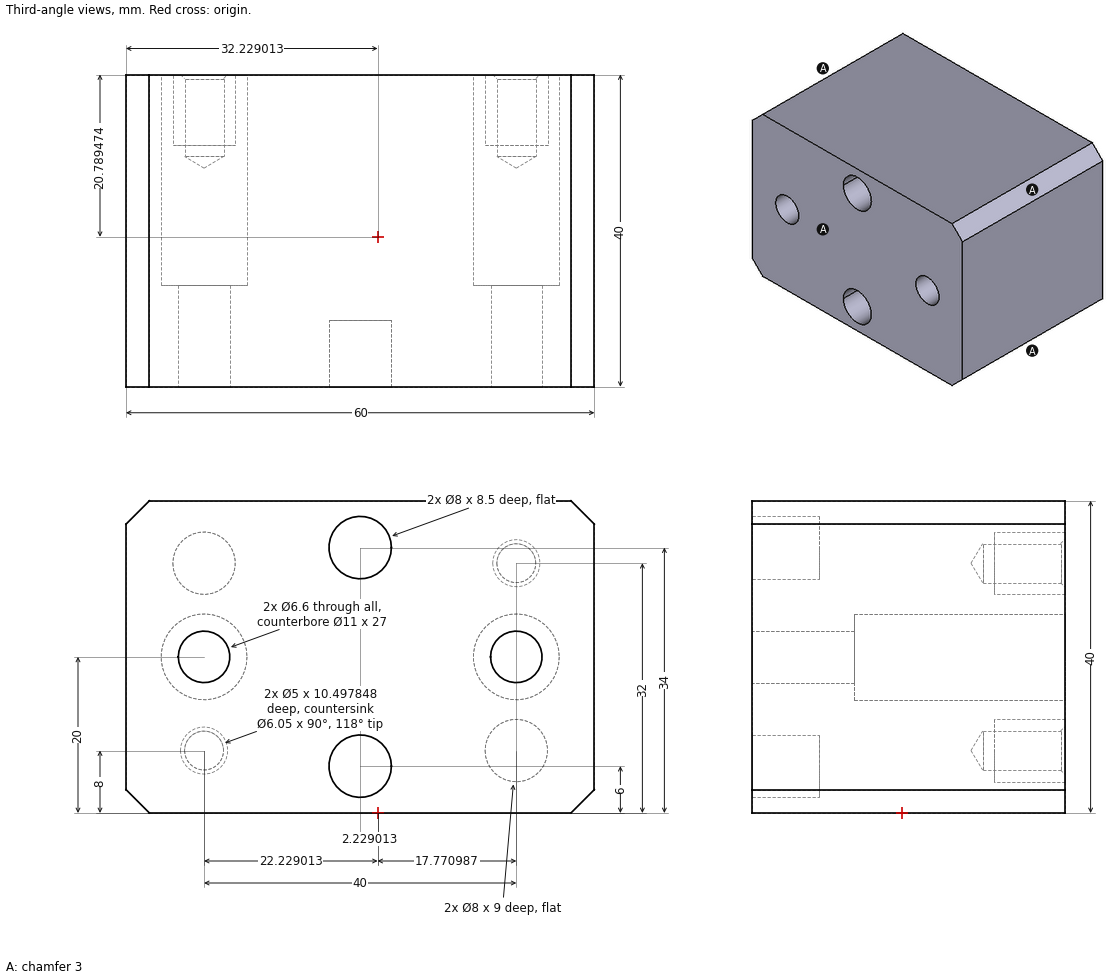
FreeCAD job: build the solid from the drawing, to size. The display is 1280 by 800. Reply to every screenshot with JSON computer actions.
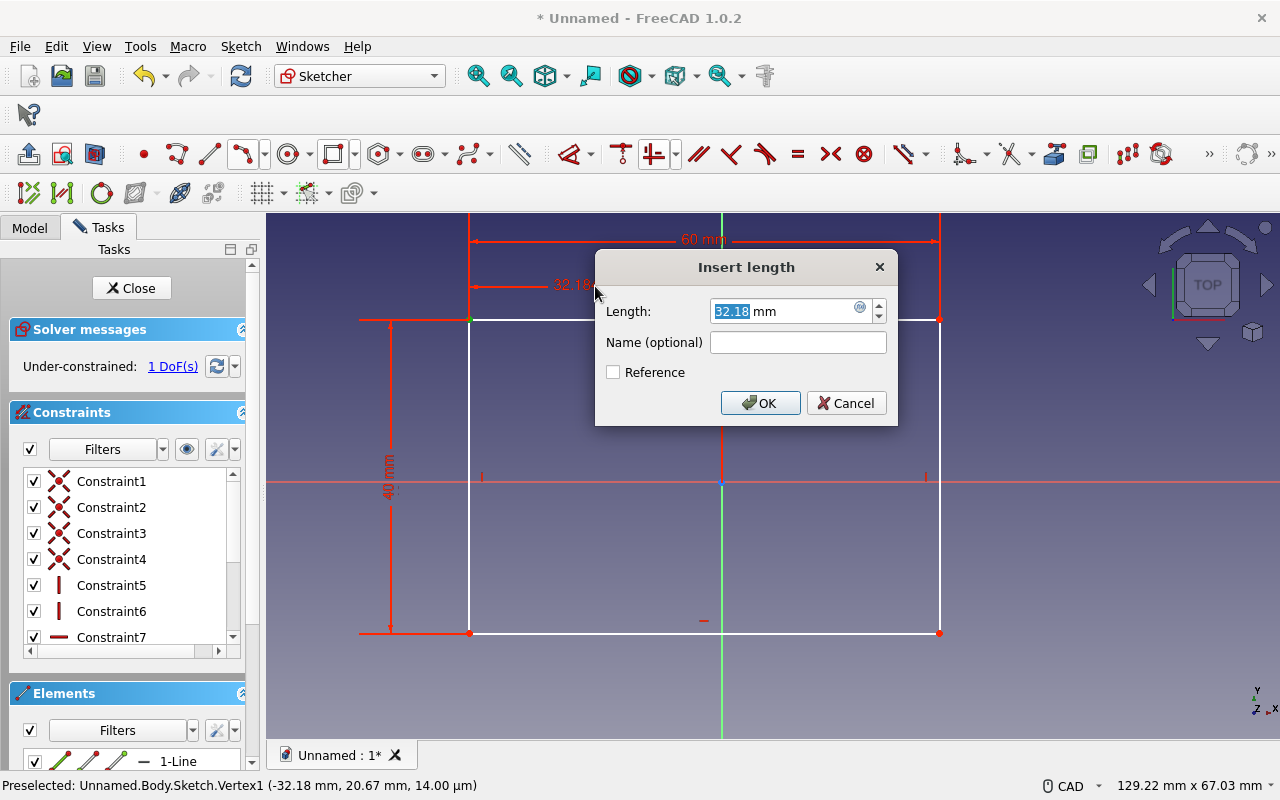
{"action": "type", "text": "32.229013"}
{"action": "key", "text": "Return"}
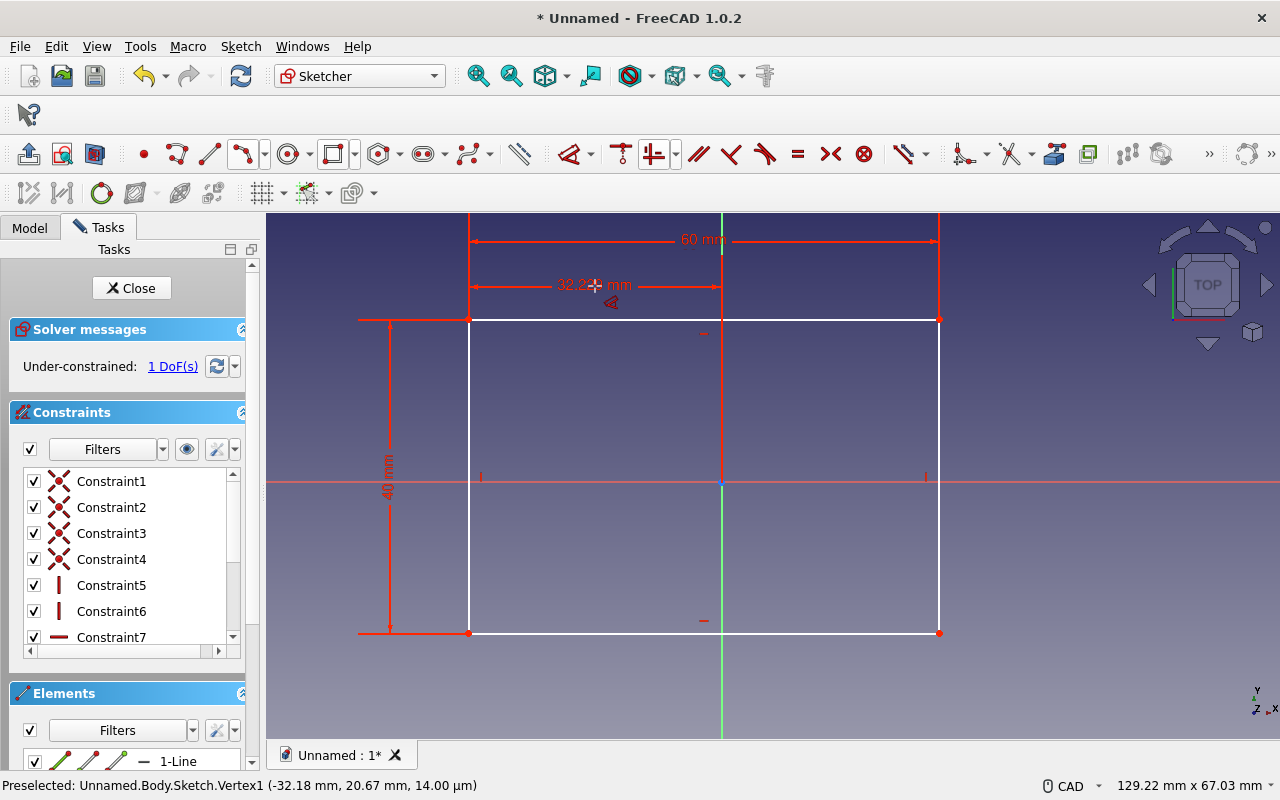
{"action": "left_click", "coordinate": [469, 320]}
{"action": "left_click", "coordinate": [435, 401]}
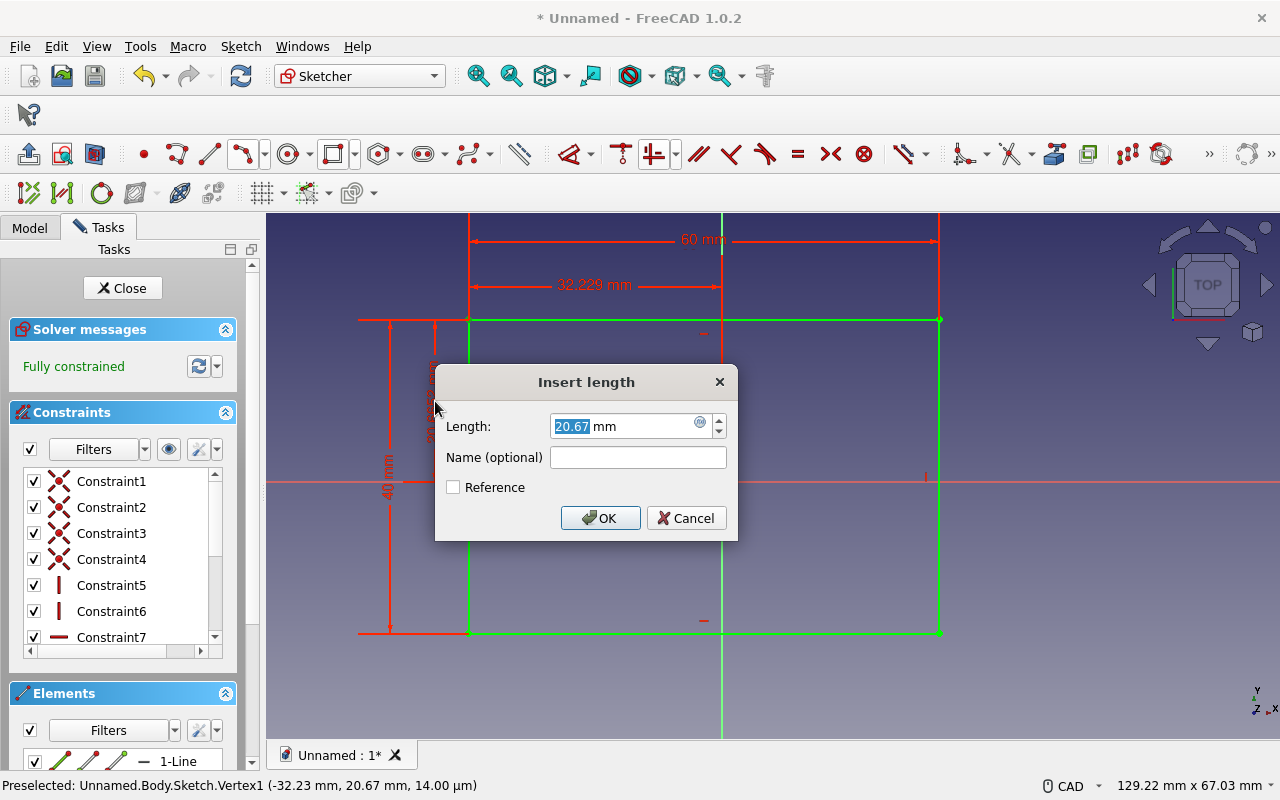
{"action": "type", "text": "20.789474"}
{"action": "key", "text": "Return"}
{"action": "key", "text": "Escape"}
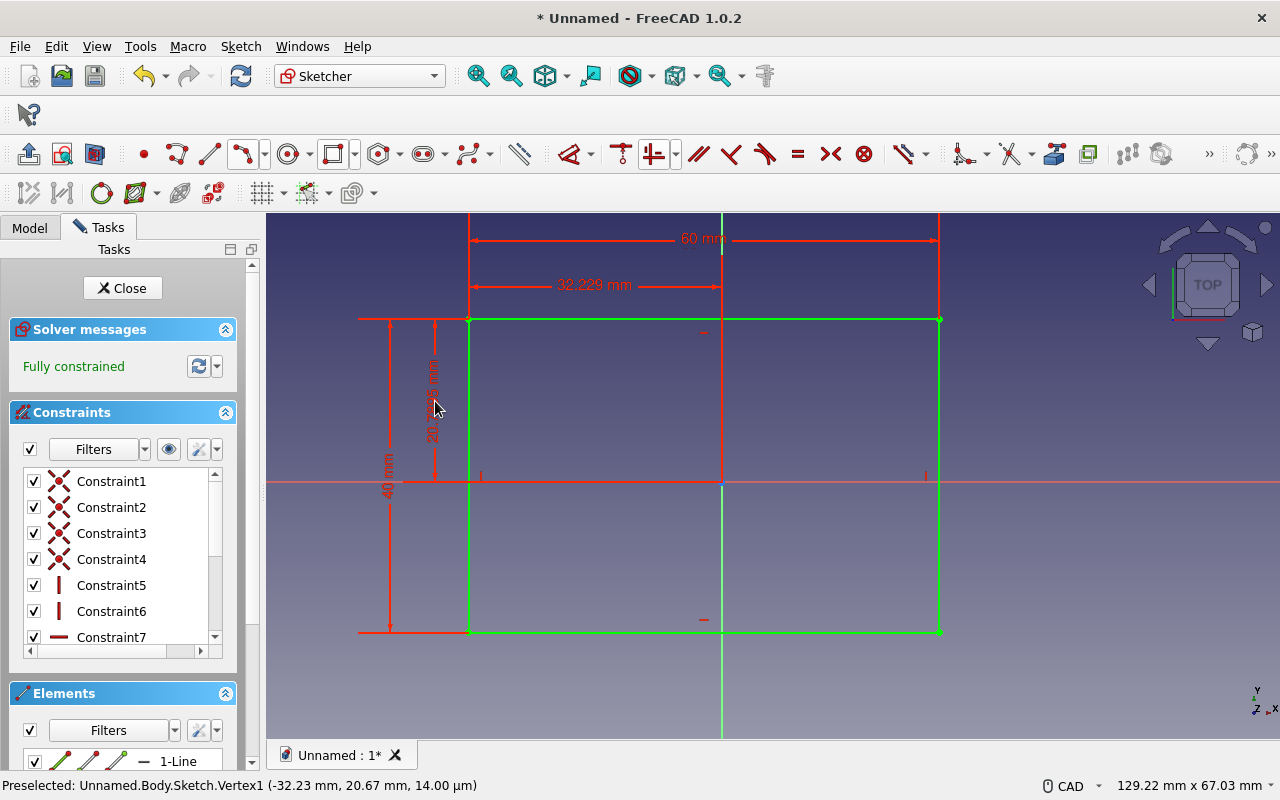
{"action": "left_click", "coordinate": [123, 288]}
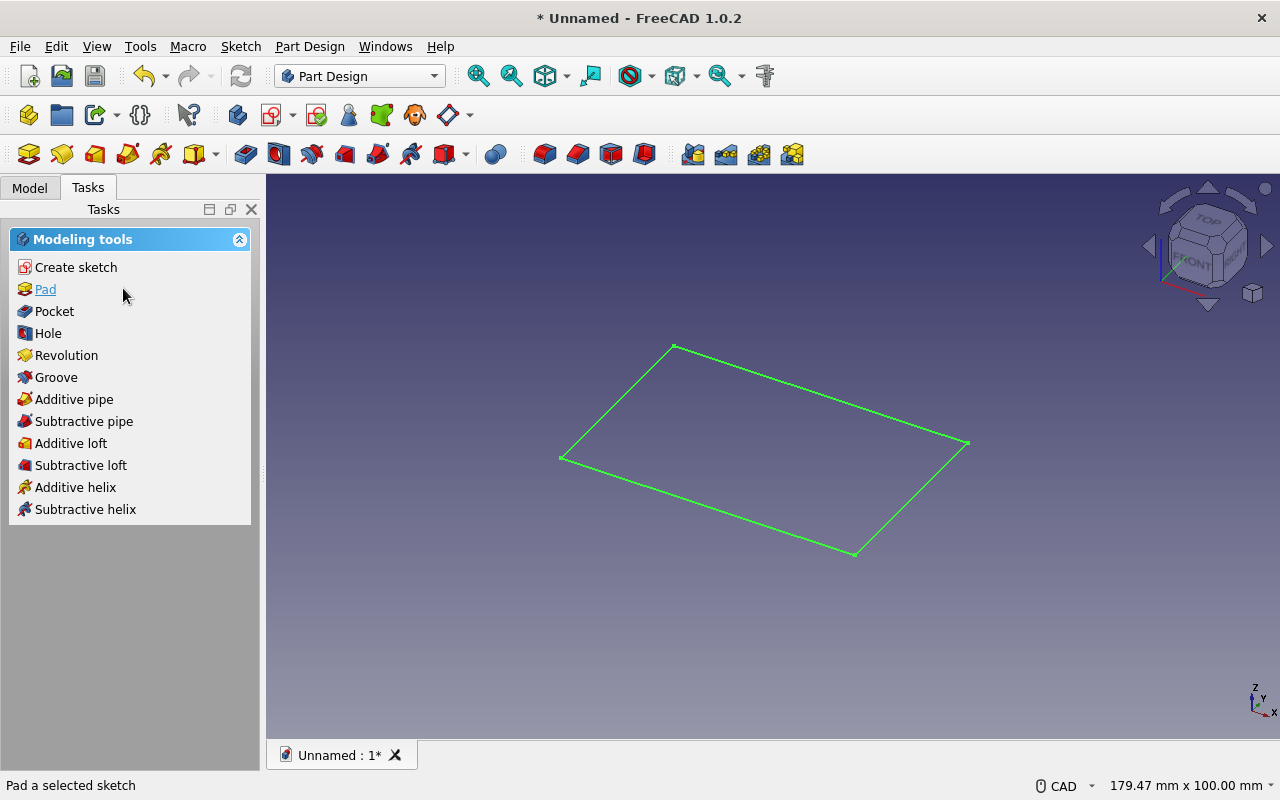
{"action": "left_click", "coordinate": [29, 154]}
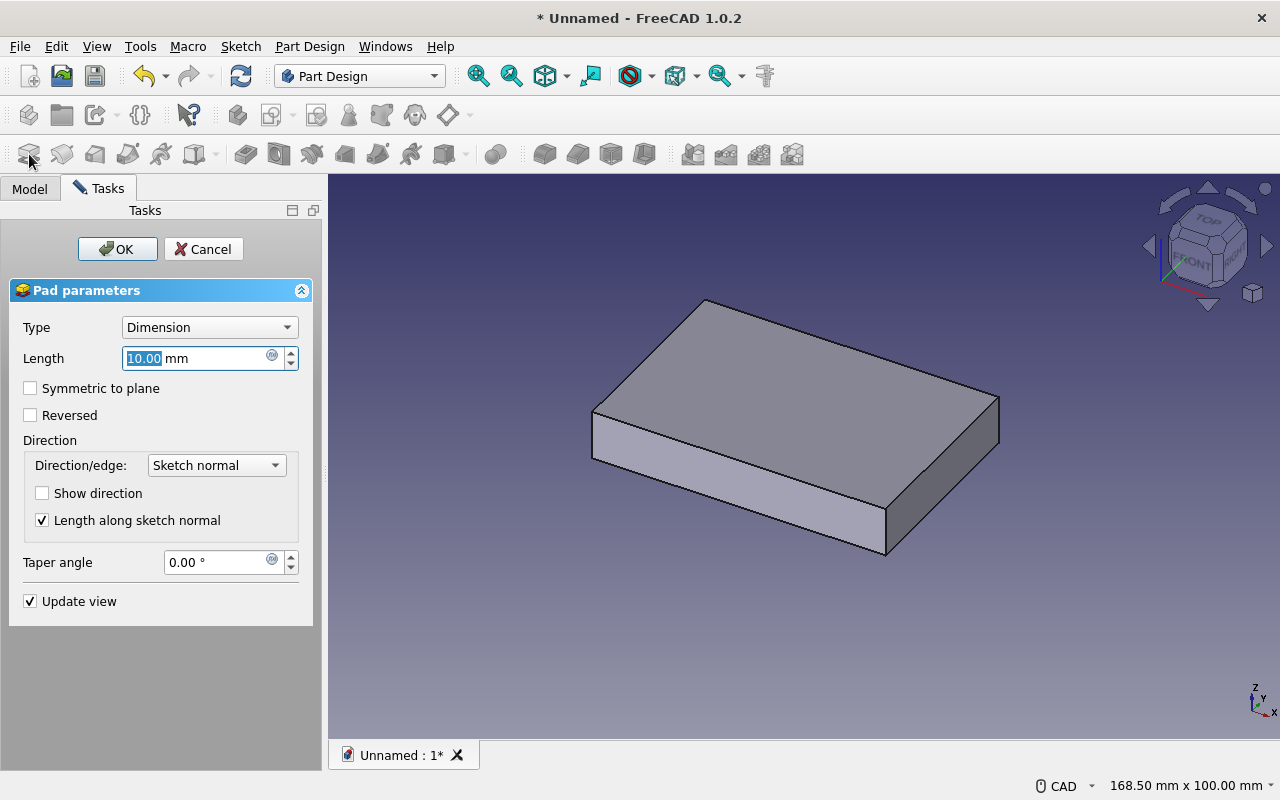
{"action": "type", "text": "40"}
{"action": "key", "text": "Tab"}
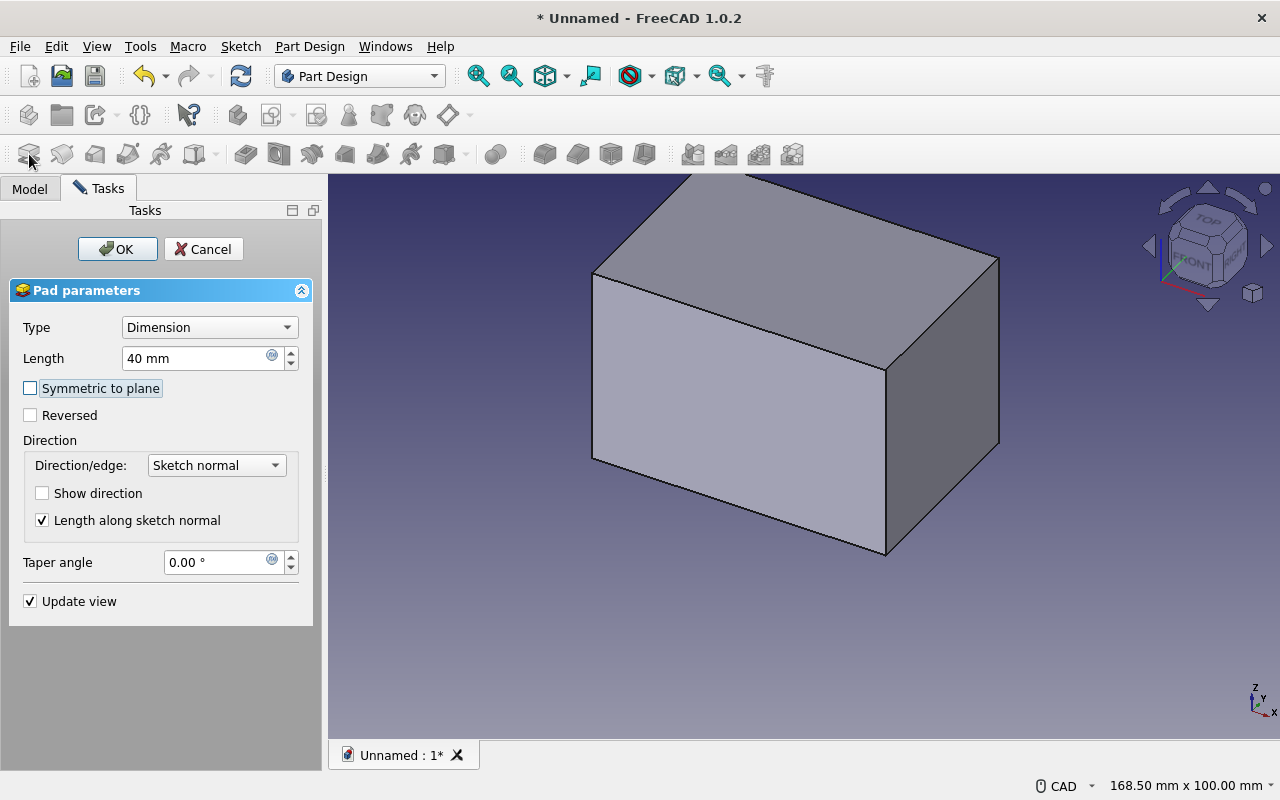
{"action": "left_click", "coordinate": [118, 249]}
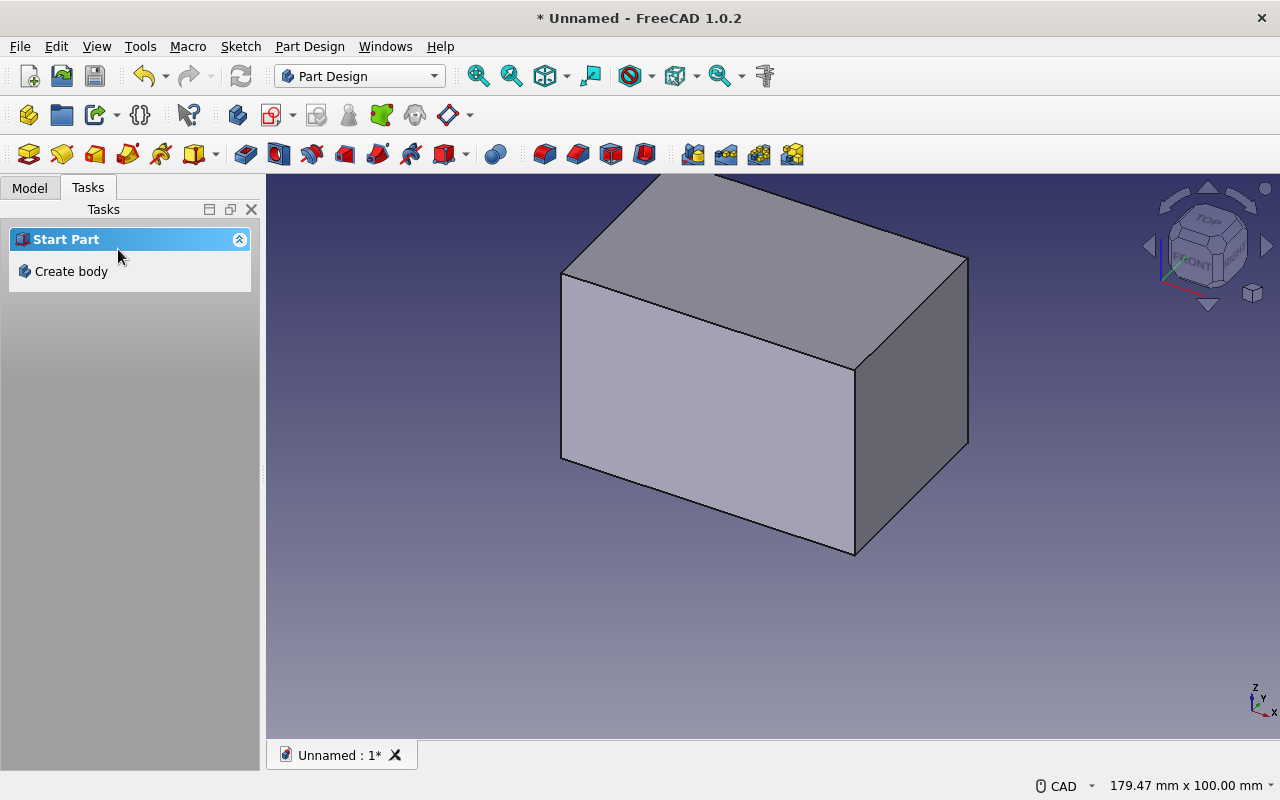
{"action": "key", "text": "v f"}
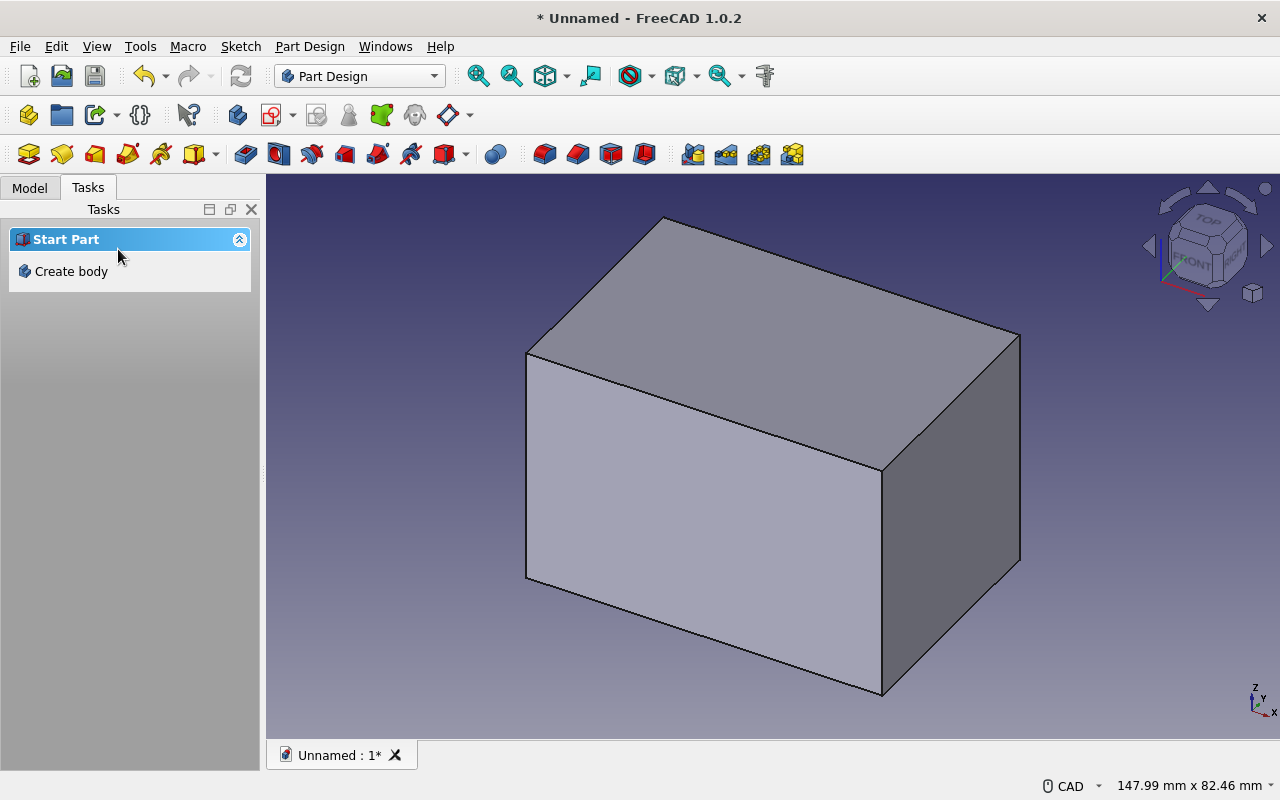
{"action": "left_click", "coordinate": [951, 402]}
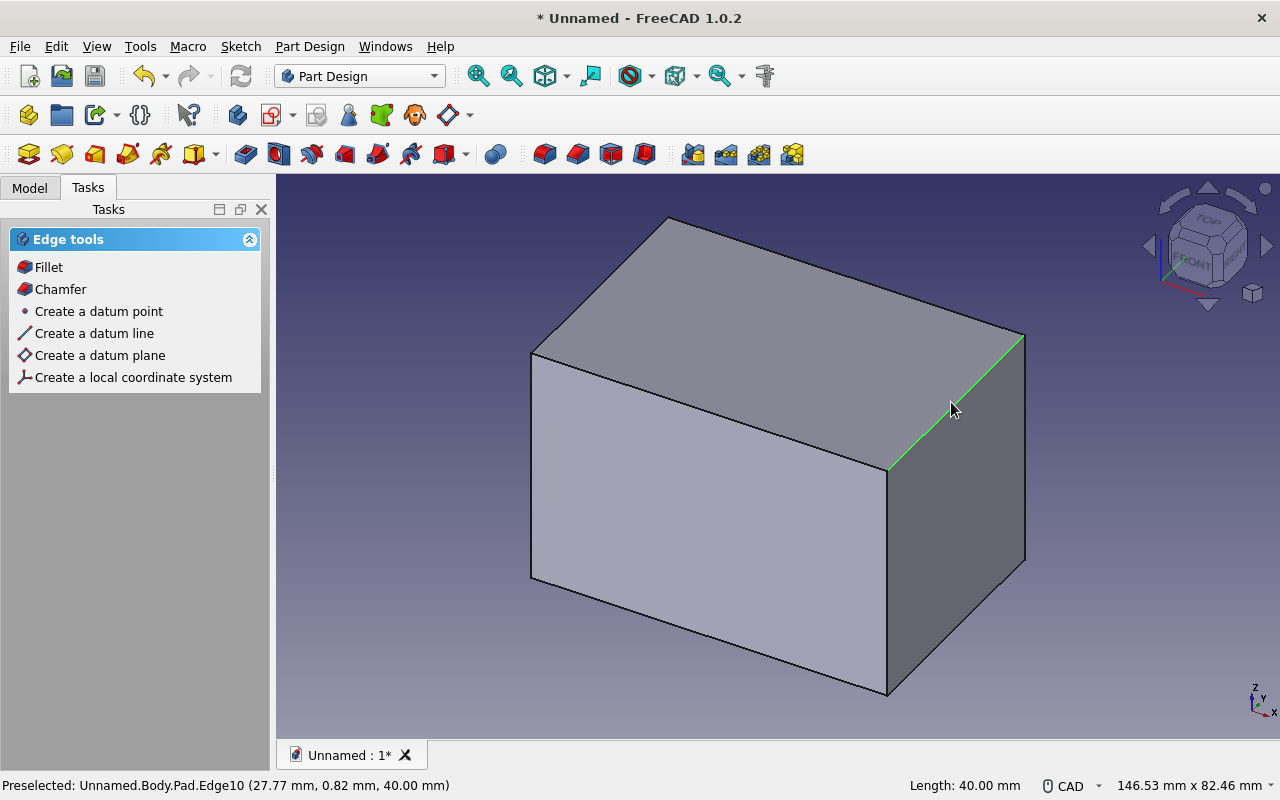
{"action": "key", "text": "0"}